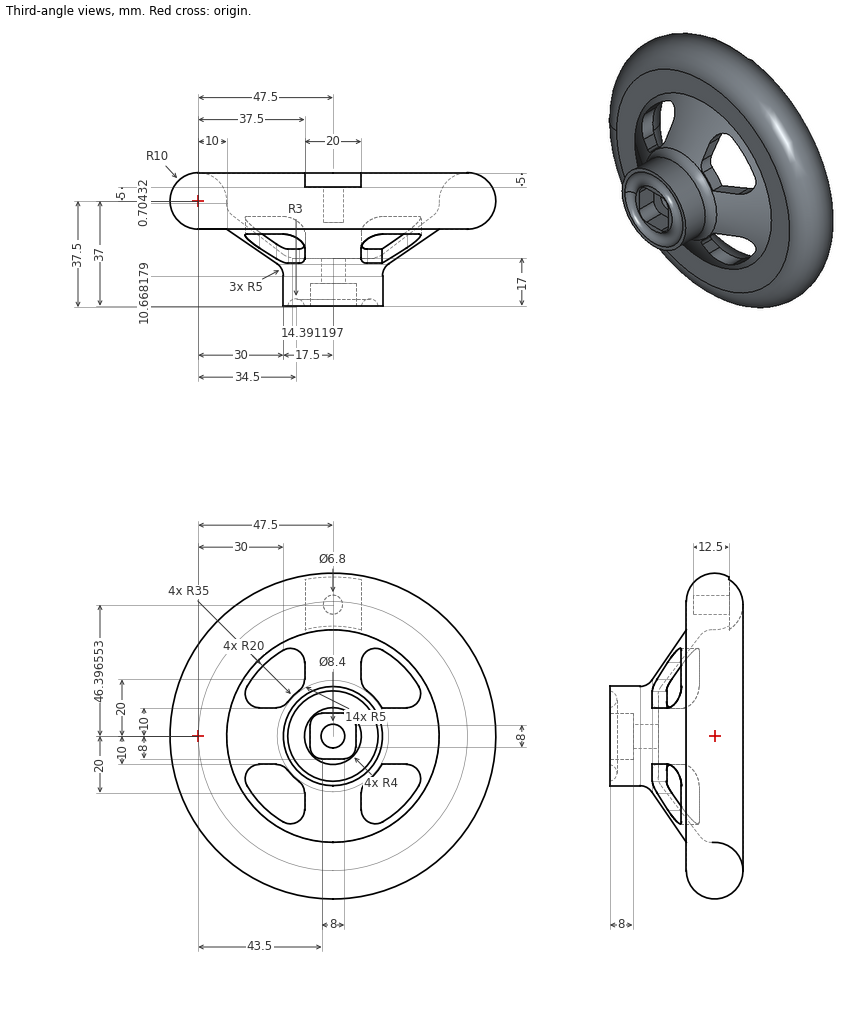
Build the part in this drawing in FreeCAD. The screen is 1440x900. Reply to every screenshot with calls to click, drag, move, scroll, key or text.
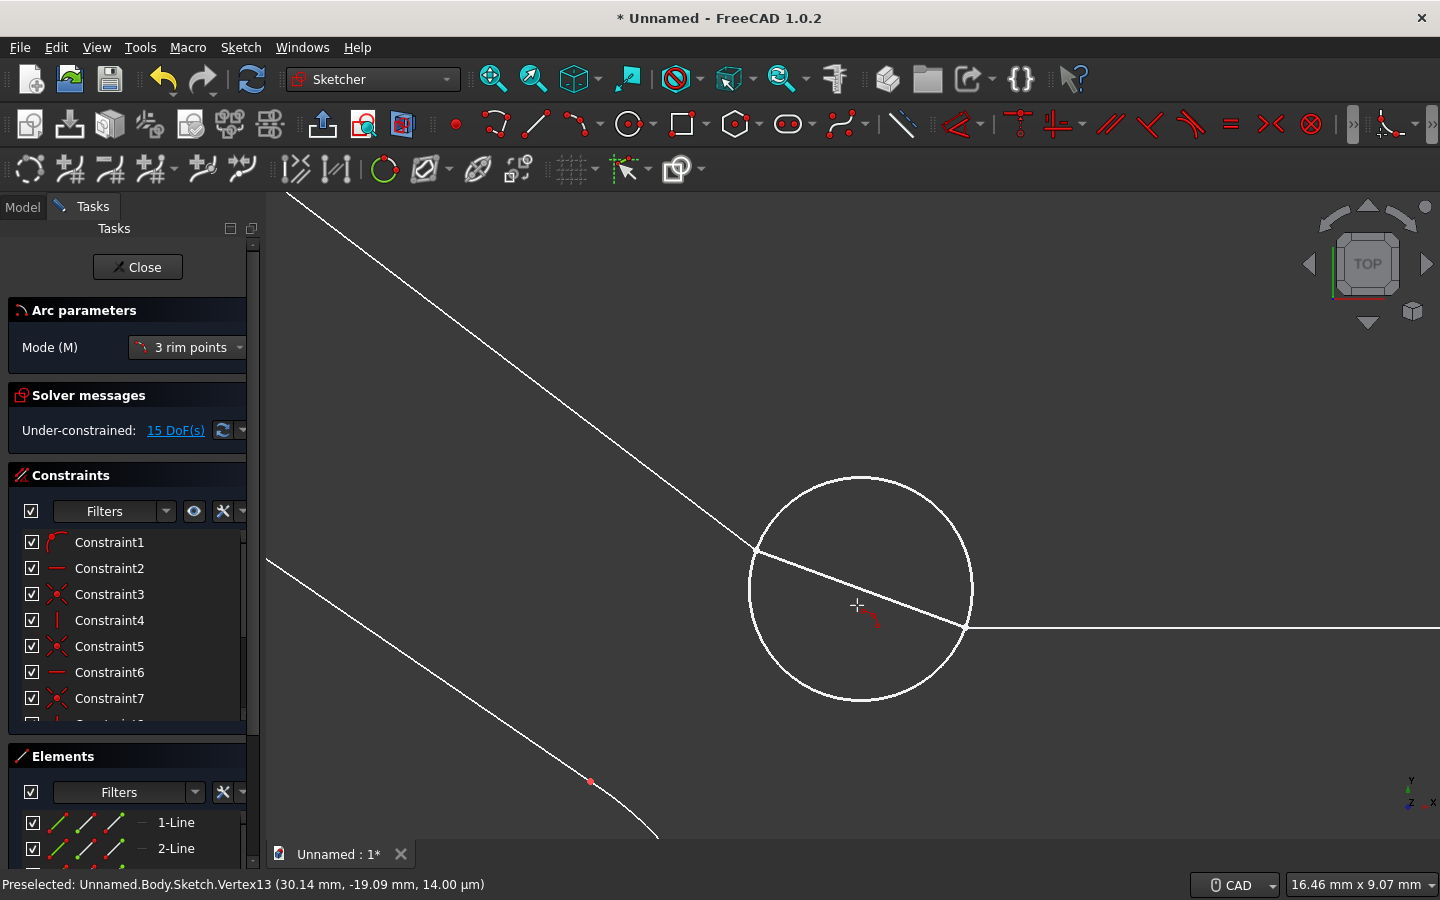
click(853, 597)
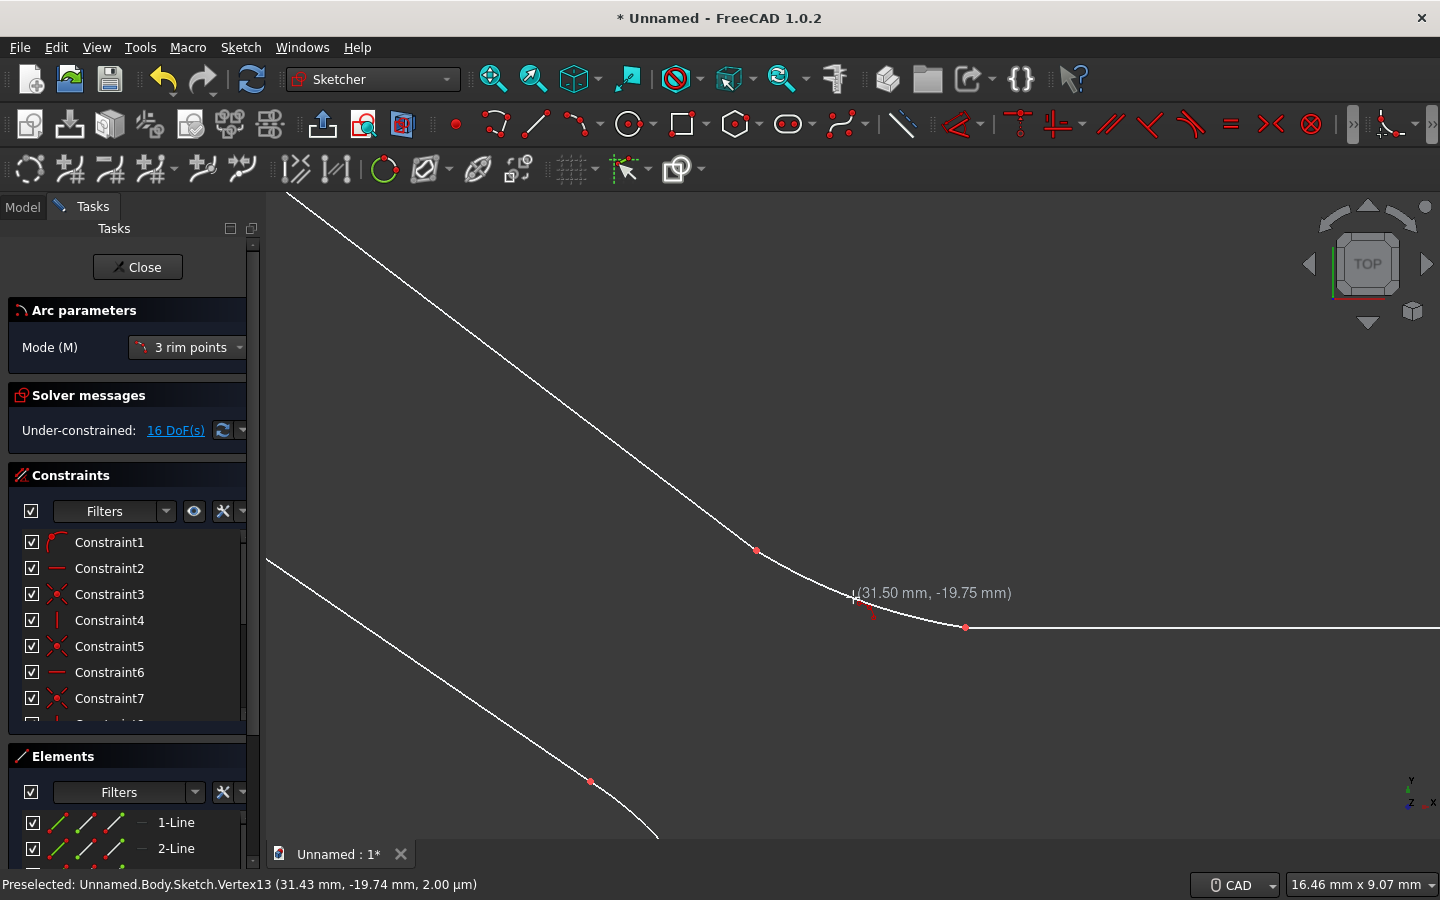
scroll(857, 605, down, 12)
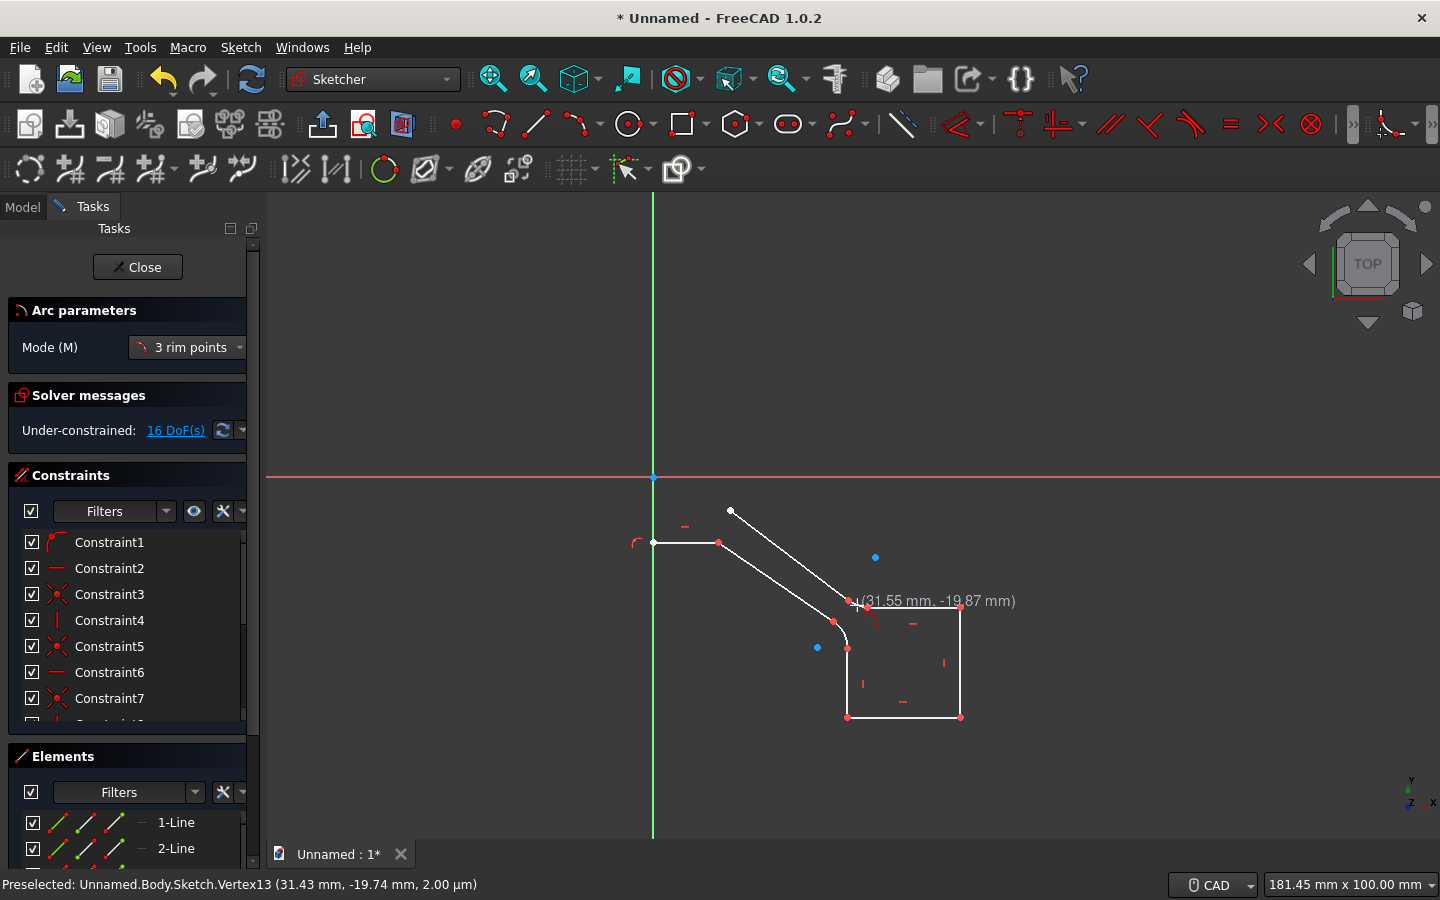
click(730, 511)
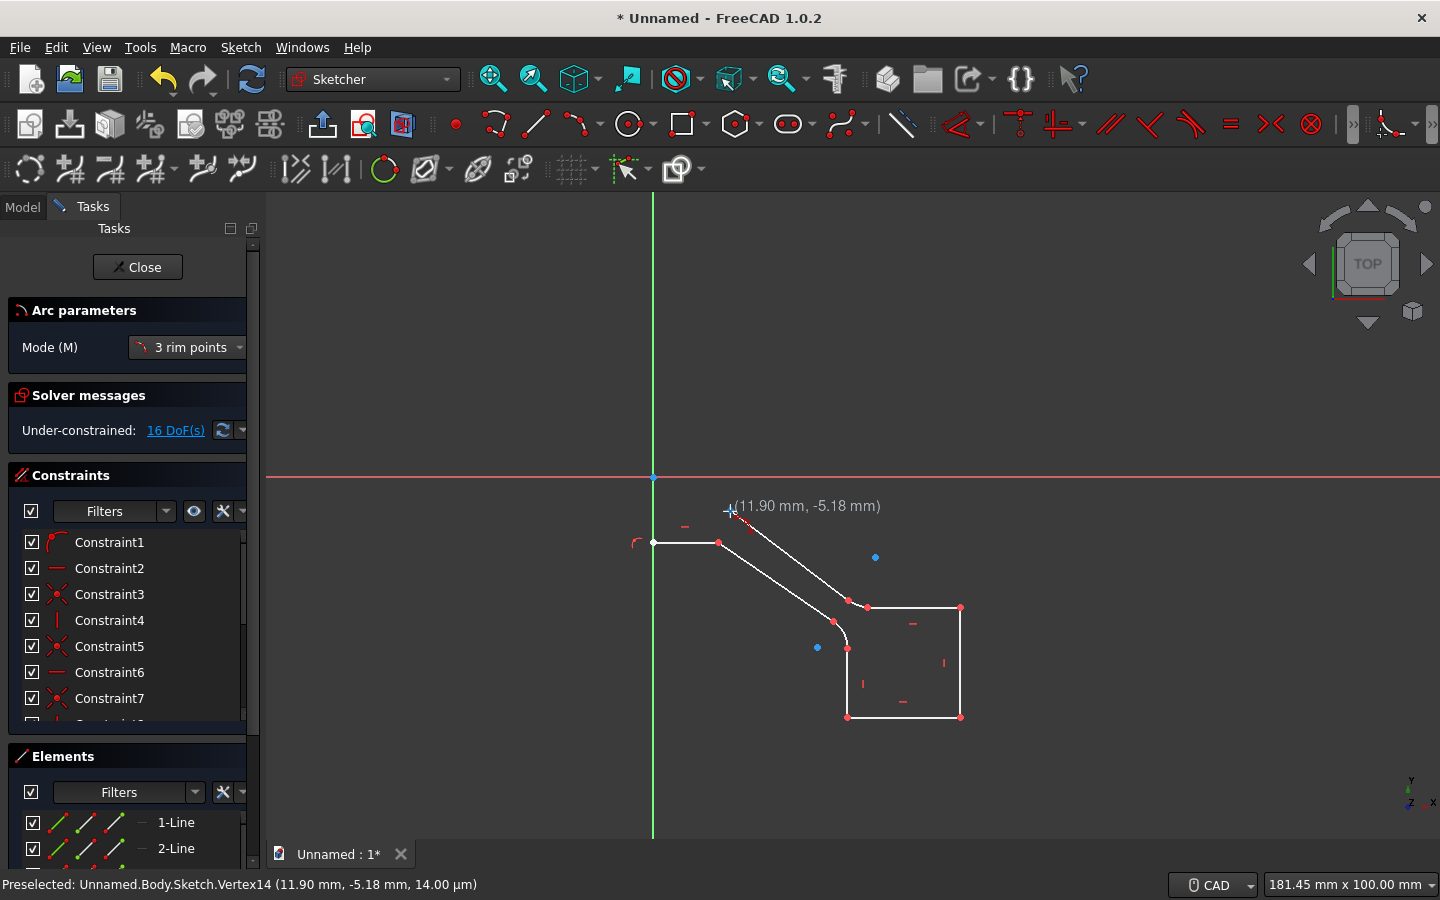
scroll(718, 482, up, 7)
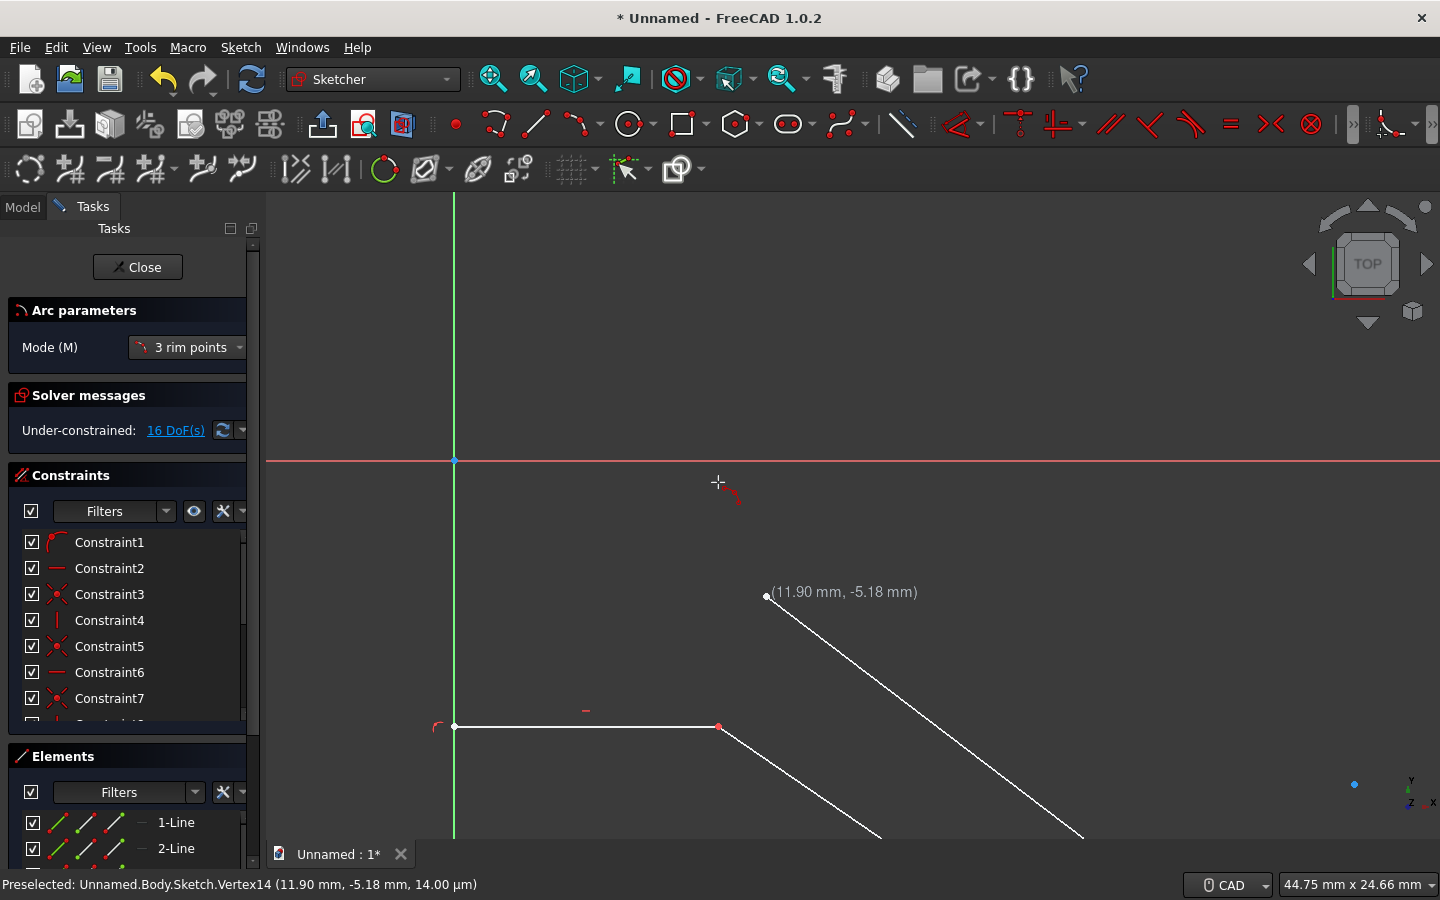
click(716, 479)
click(727, 542)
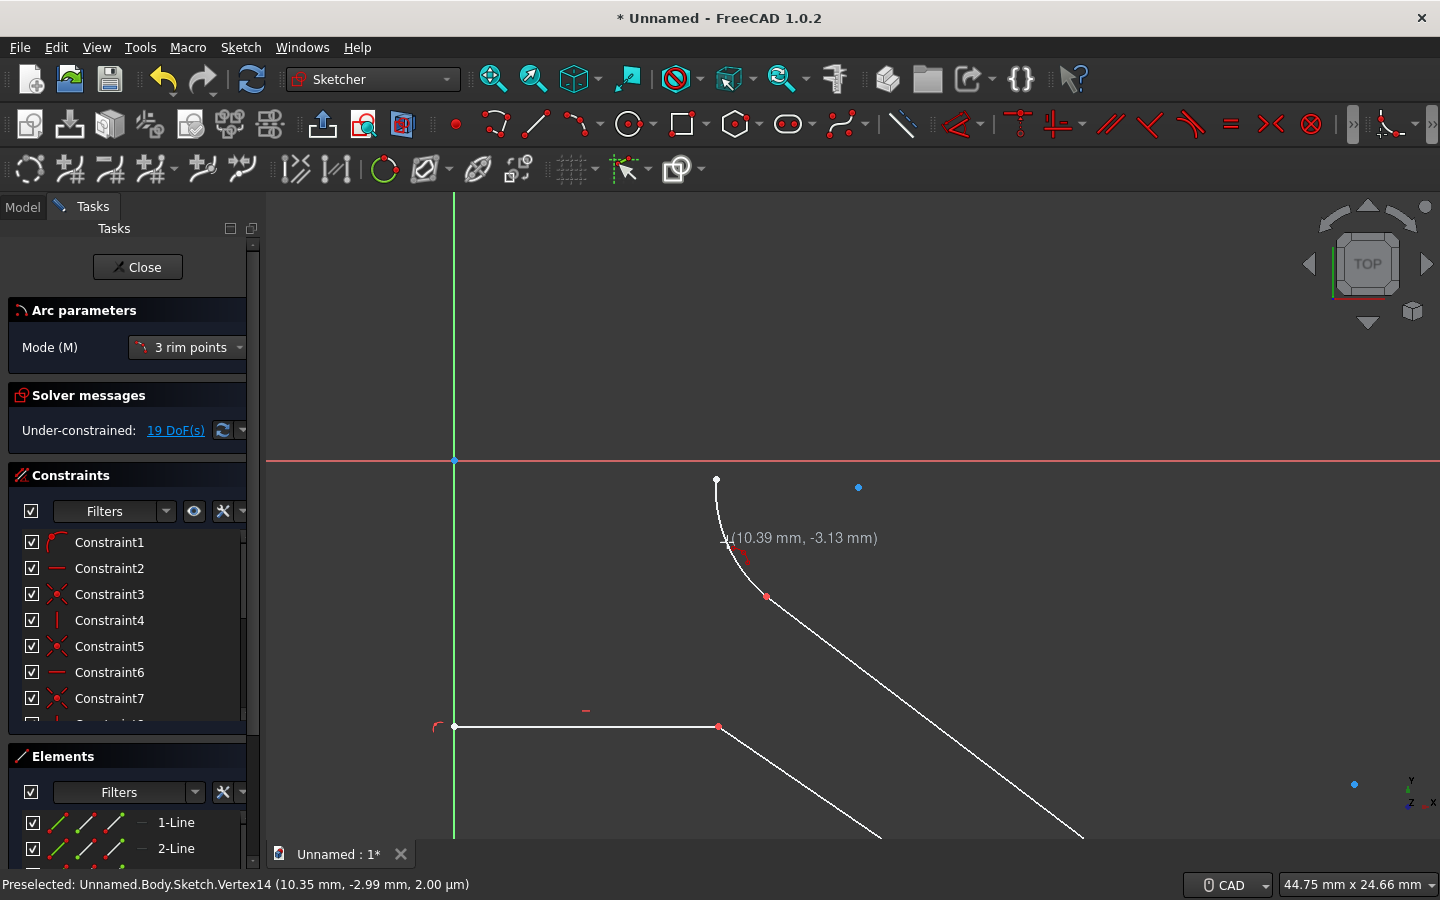
click(716, 480)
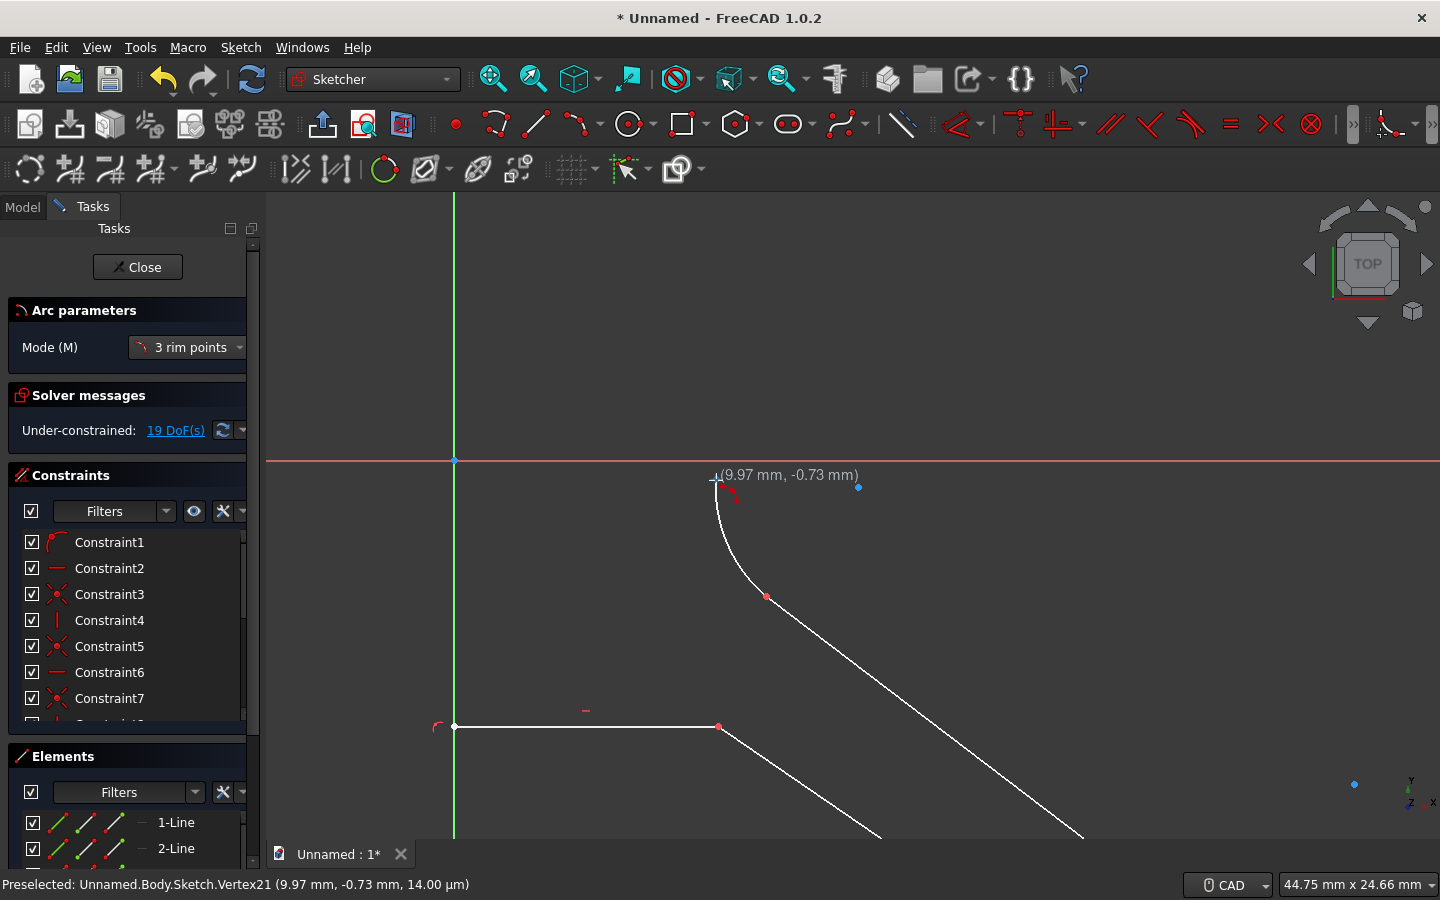
scroll(718, 482, down, 7)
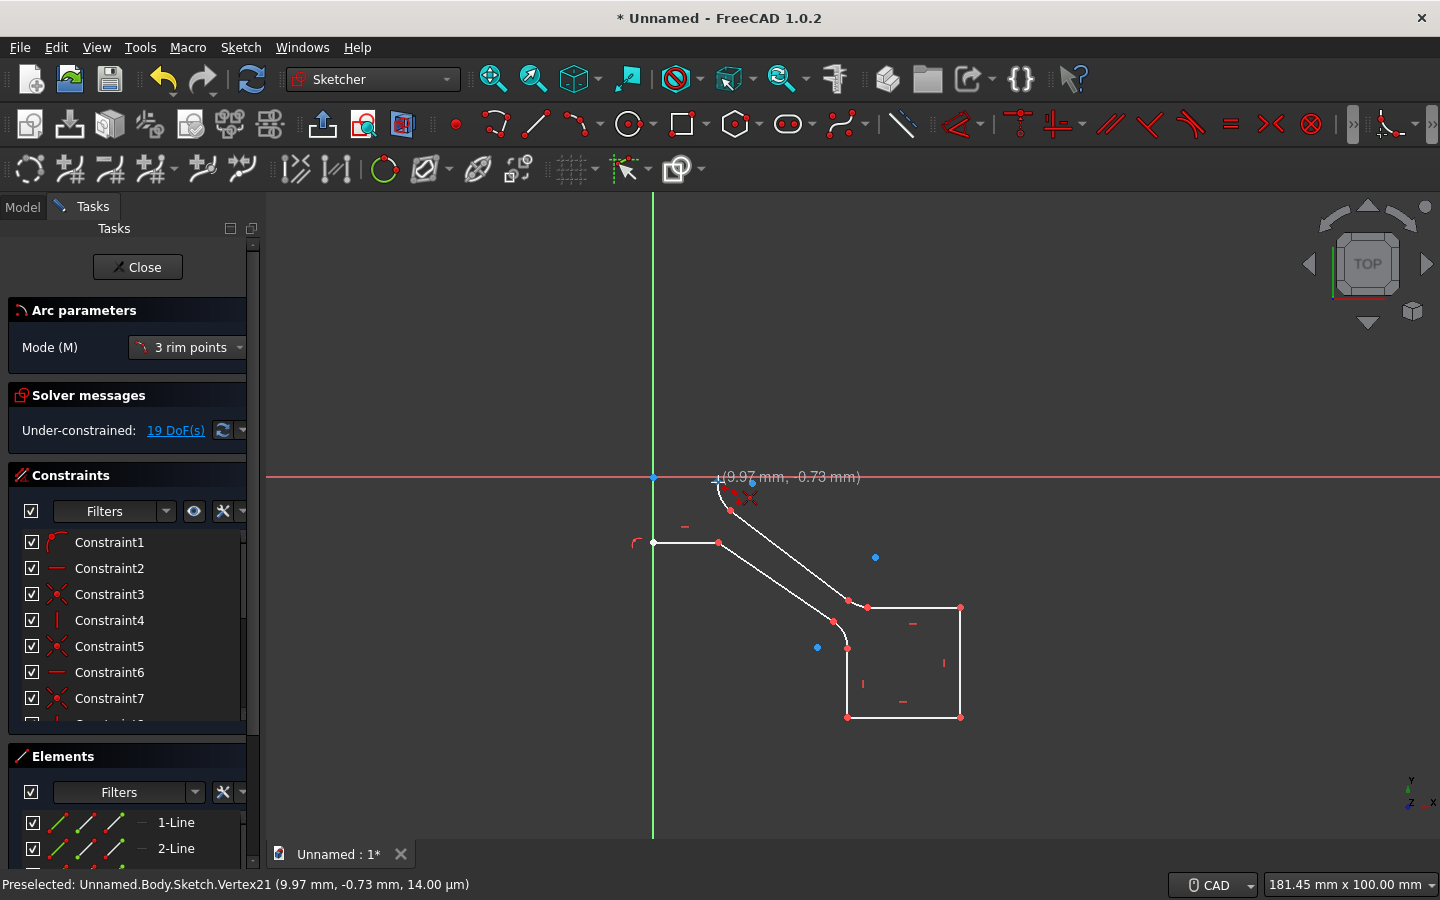
click(653, 543)
click(609, 430)